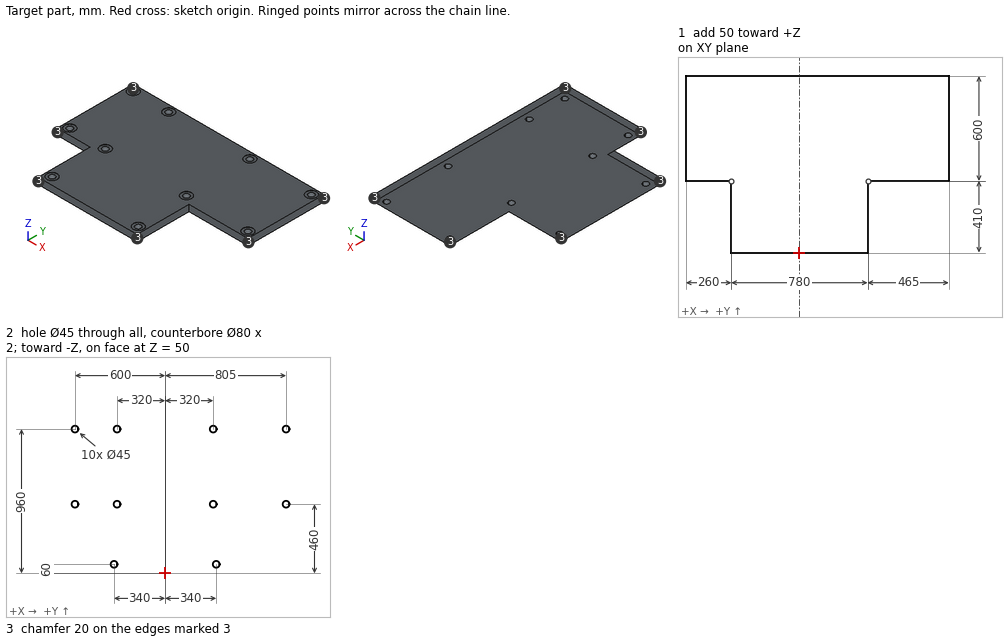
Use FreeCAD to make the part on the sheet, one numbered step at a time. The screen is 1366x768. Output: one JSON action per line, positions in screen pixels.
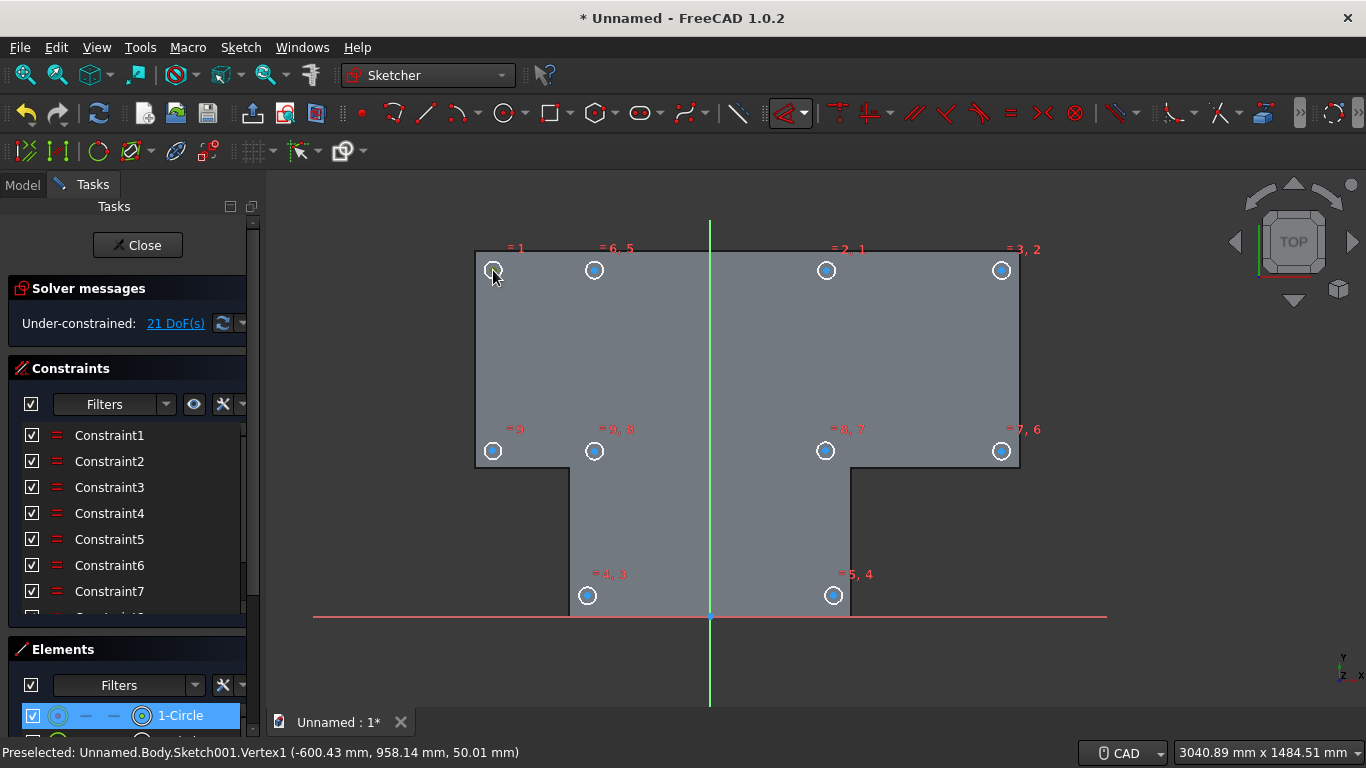
{"action": "left_click", "coordinate": [827, 271]}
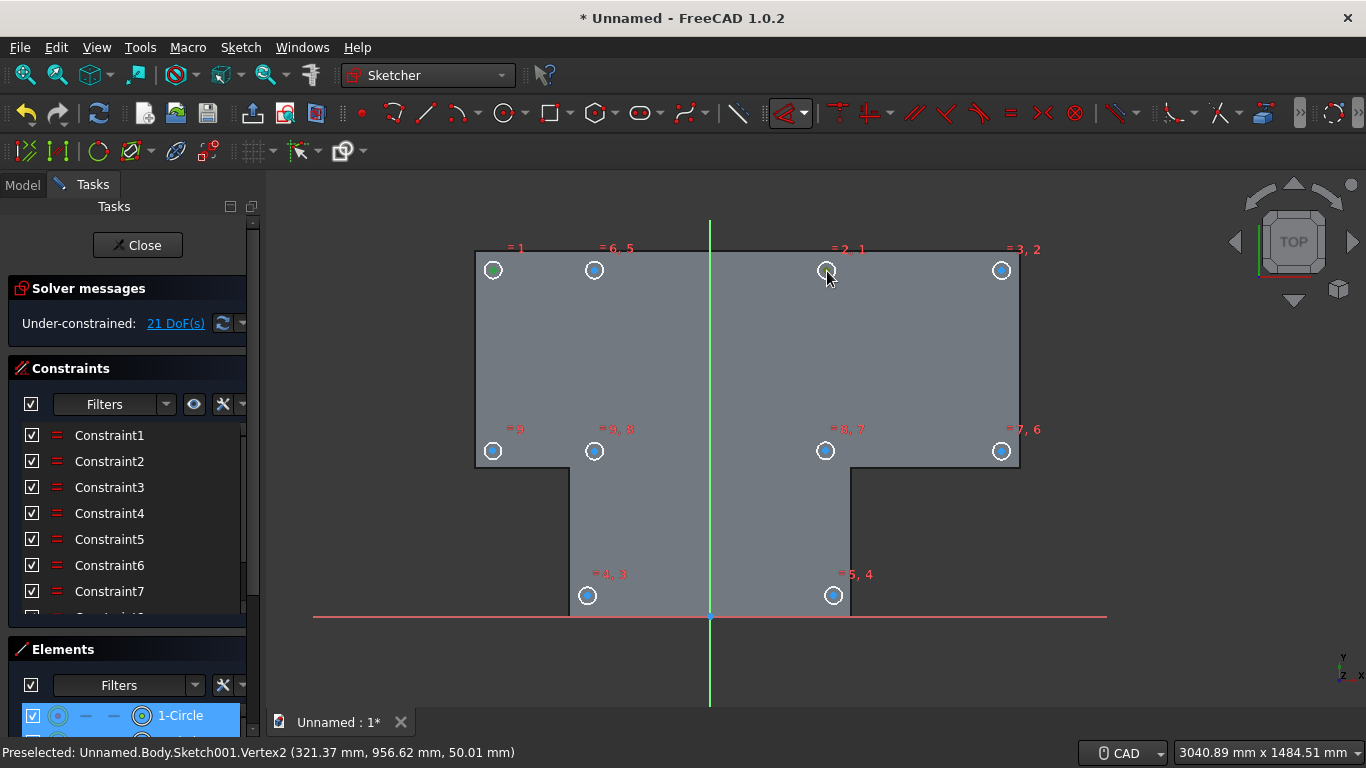
{"action": "left_click", "coordinate": [892, 114]}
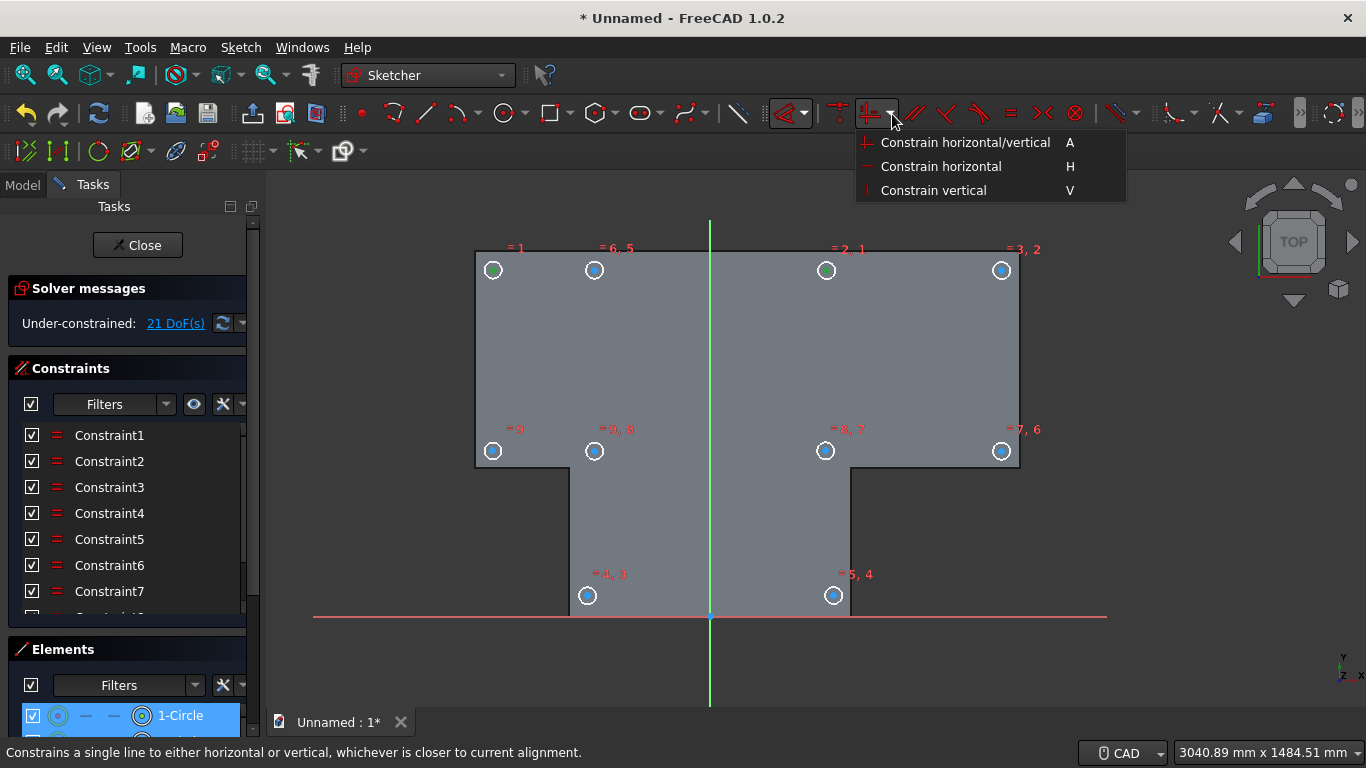
{"action": "left_click", "coordinate": [991, 166]}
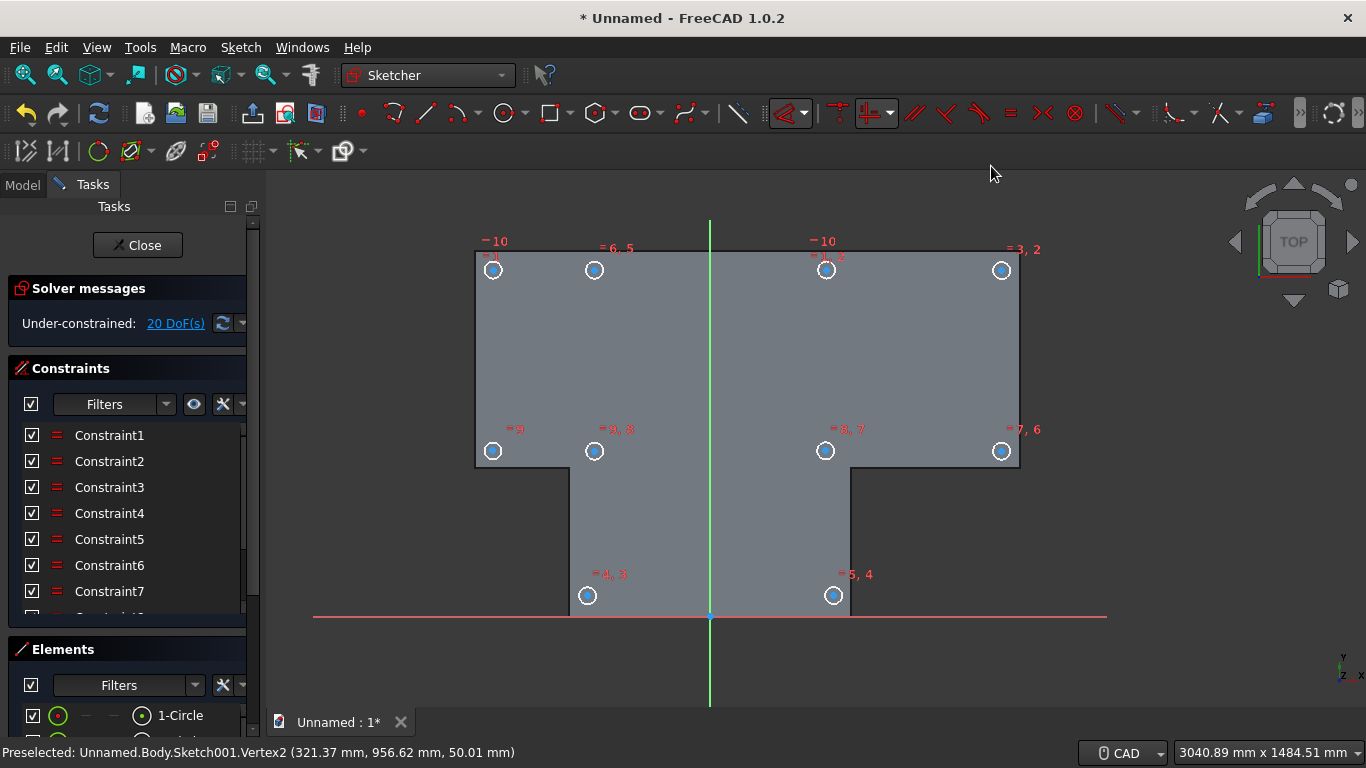
{"action": "left_click", "coordinate": [827, 270]}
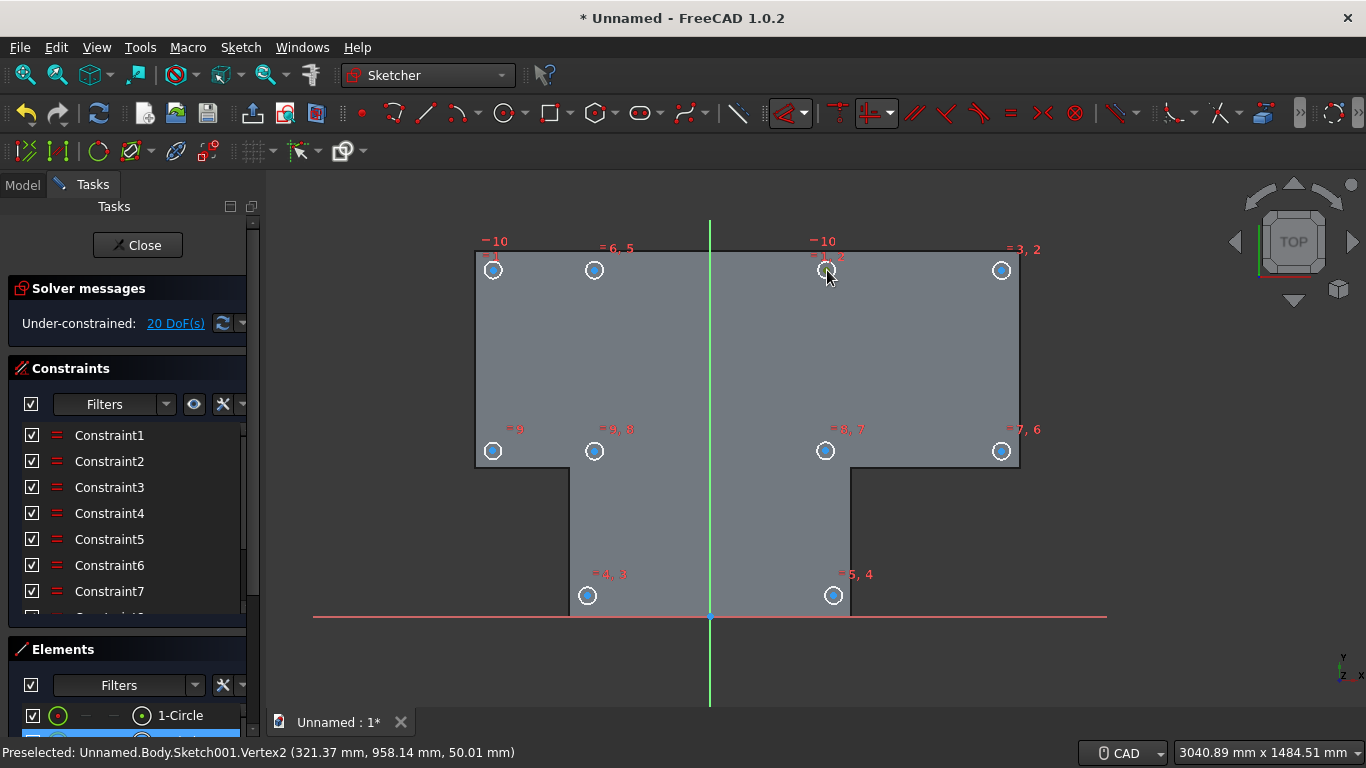
{"action": "left_click", "coordinate": [1002, 271]}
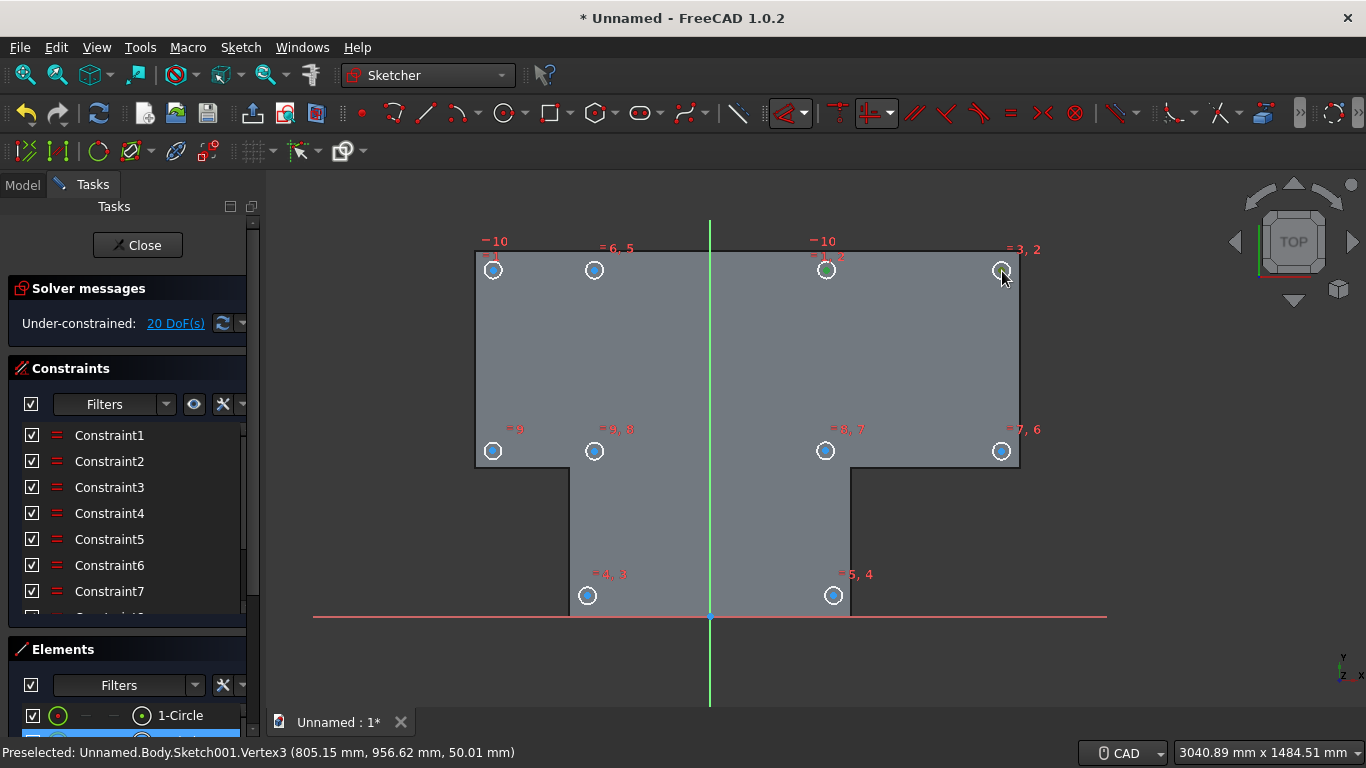
{"action": "left_click", "coordinate": [892, 114]}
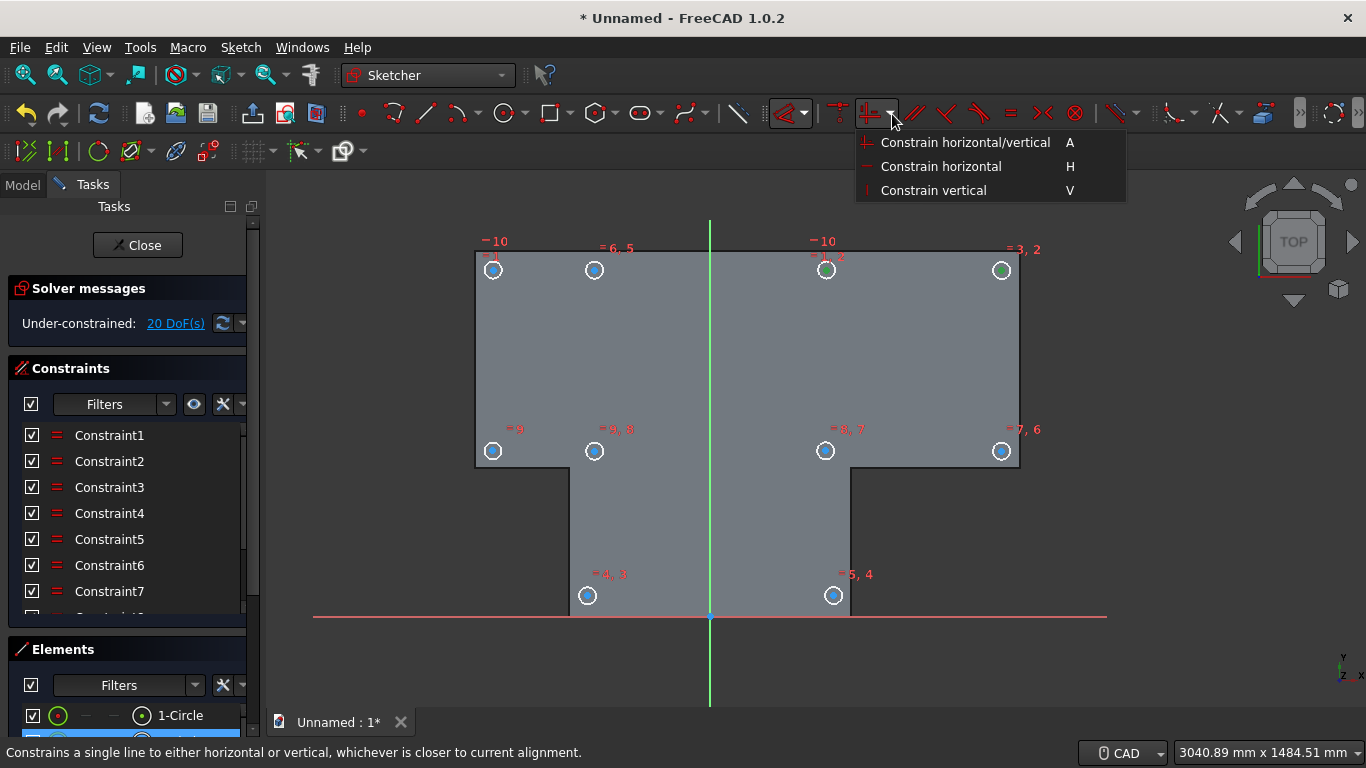
{"action": "left_click", "coordinate": [991, 166]}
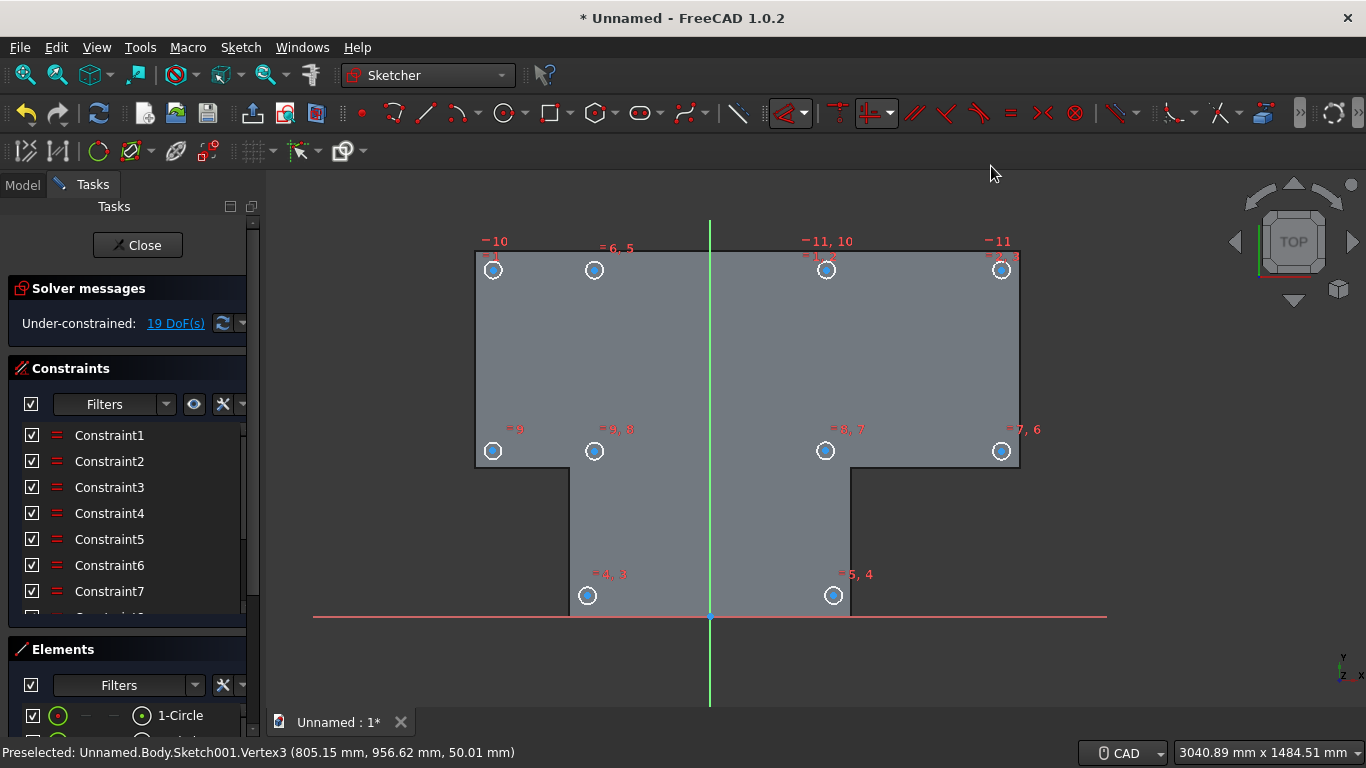
{"action": "left_click", "coordinate": [588, 596]}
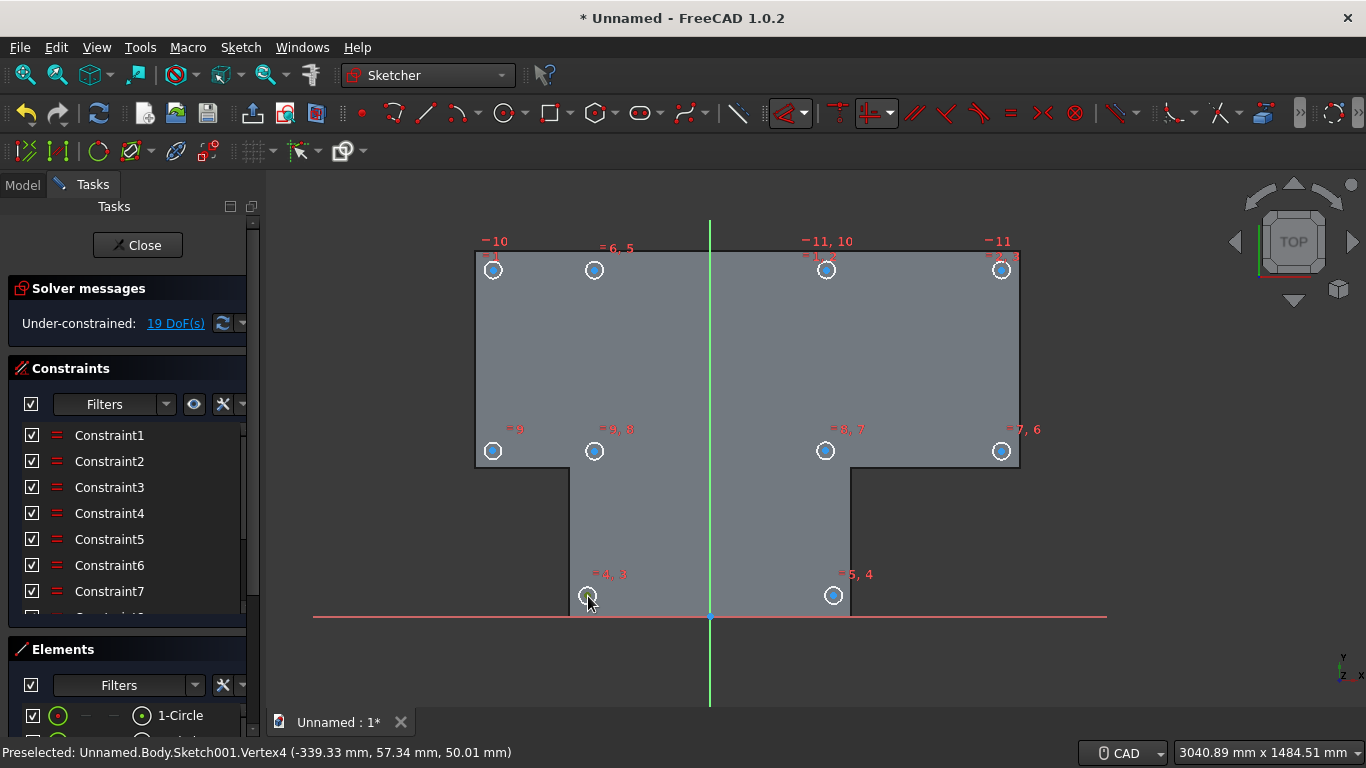
{"action": "left_click", "coordinate": [834, 596]}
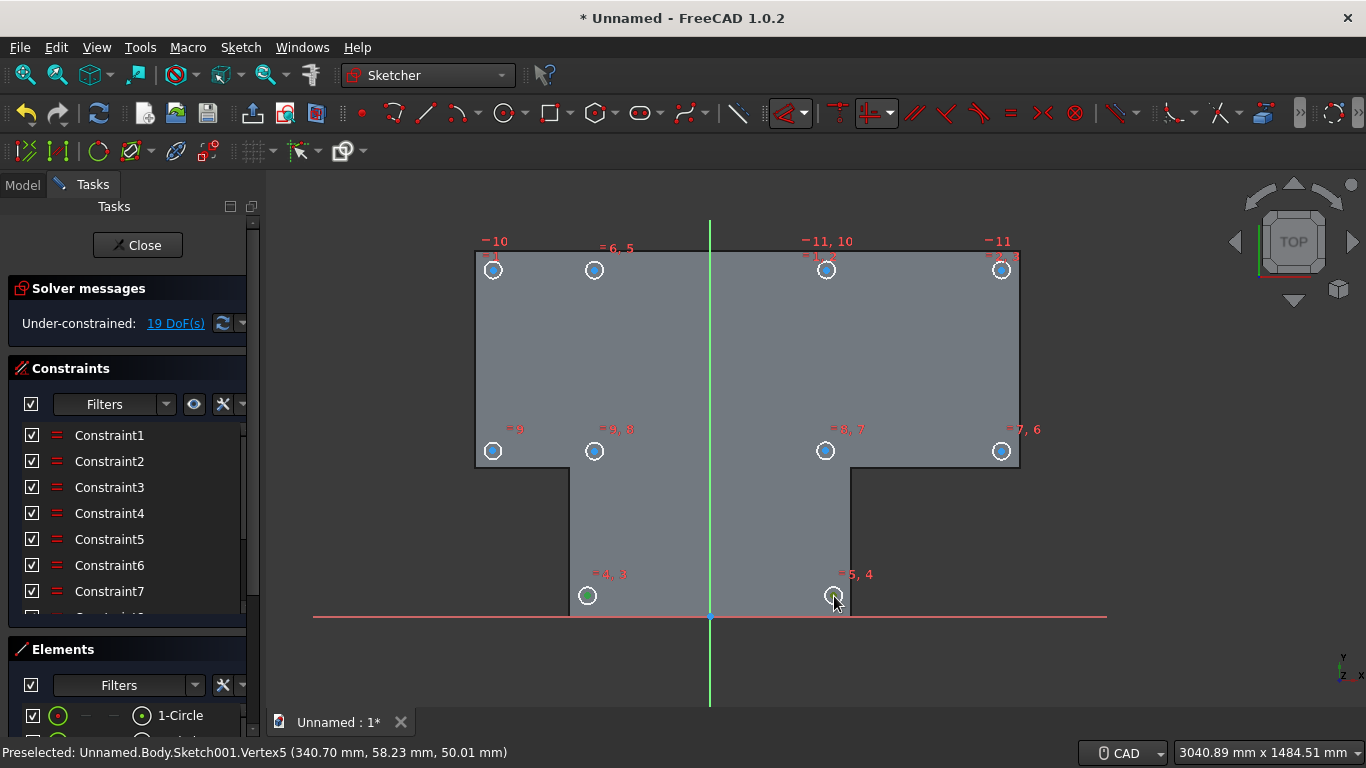
{"action": "key", "text": "h"}